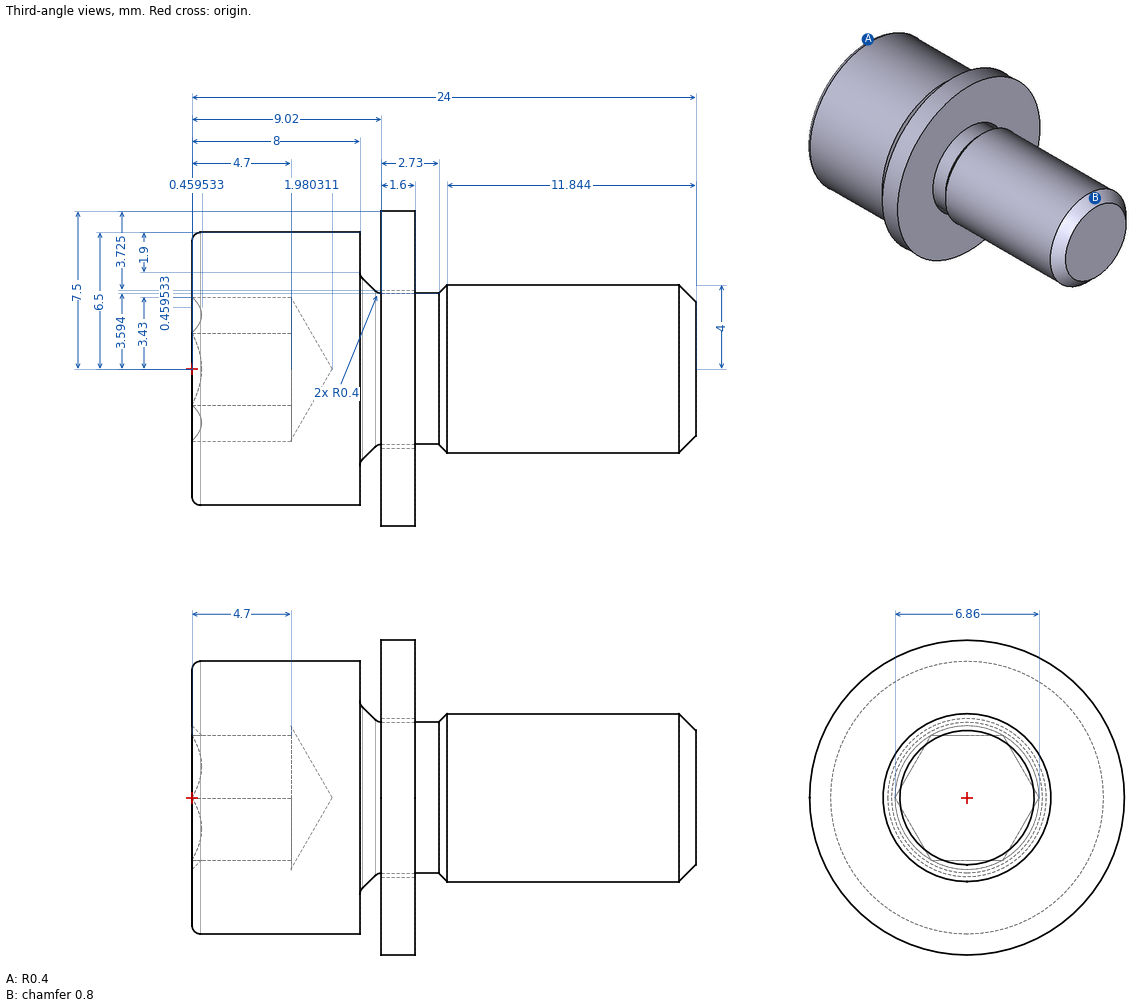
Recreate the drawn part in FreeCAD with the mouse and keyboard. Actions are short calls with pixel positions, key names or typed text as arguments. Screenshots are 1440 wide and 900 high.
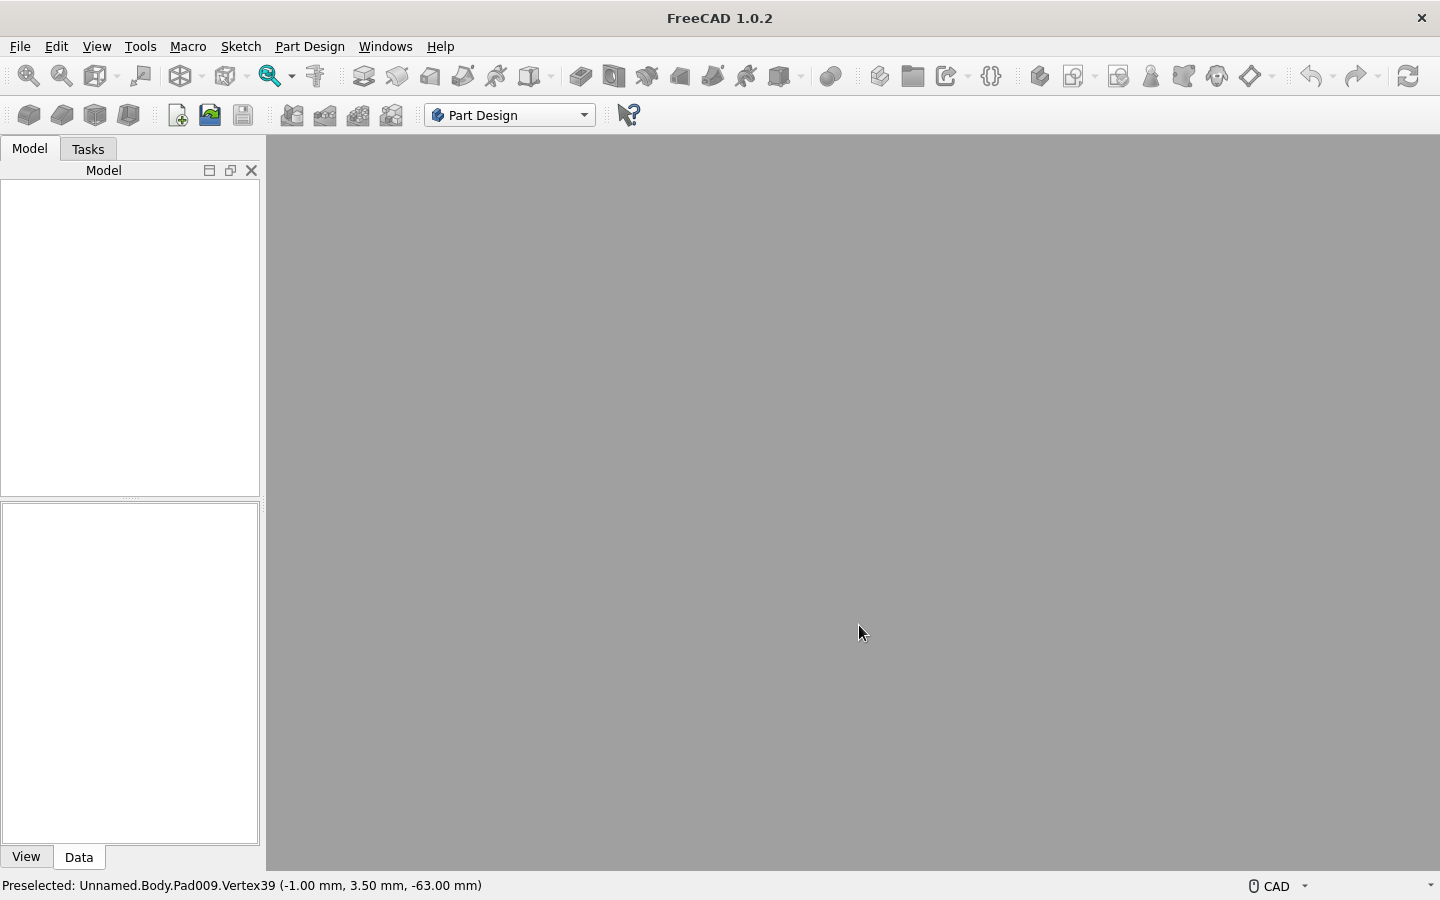
click(177, 116)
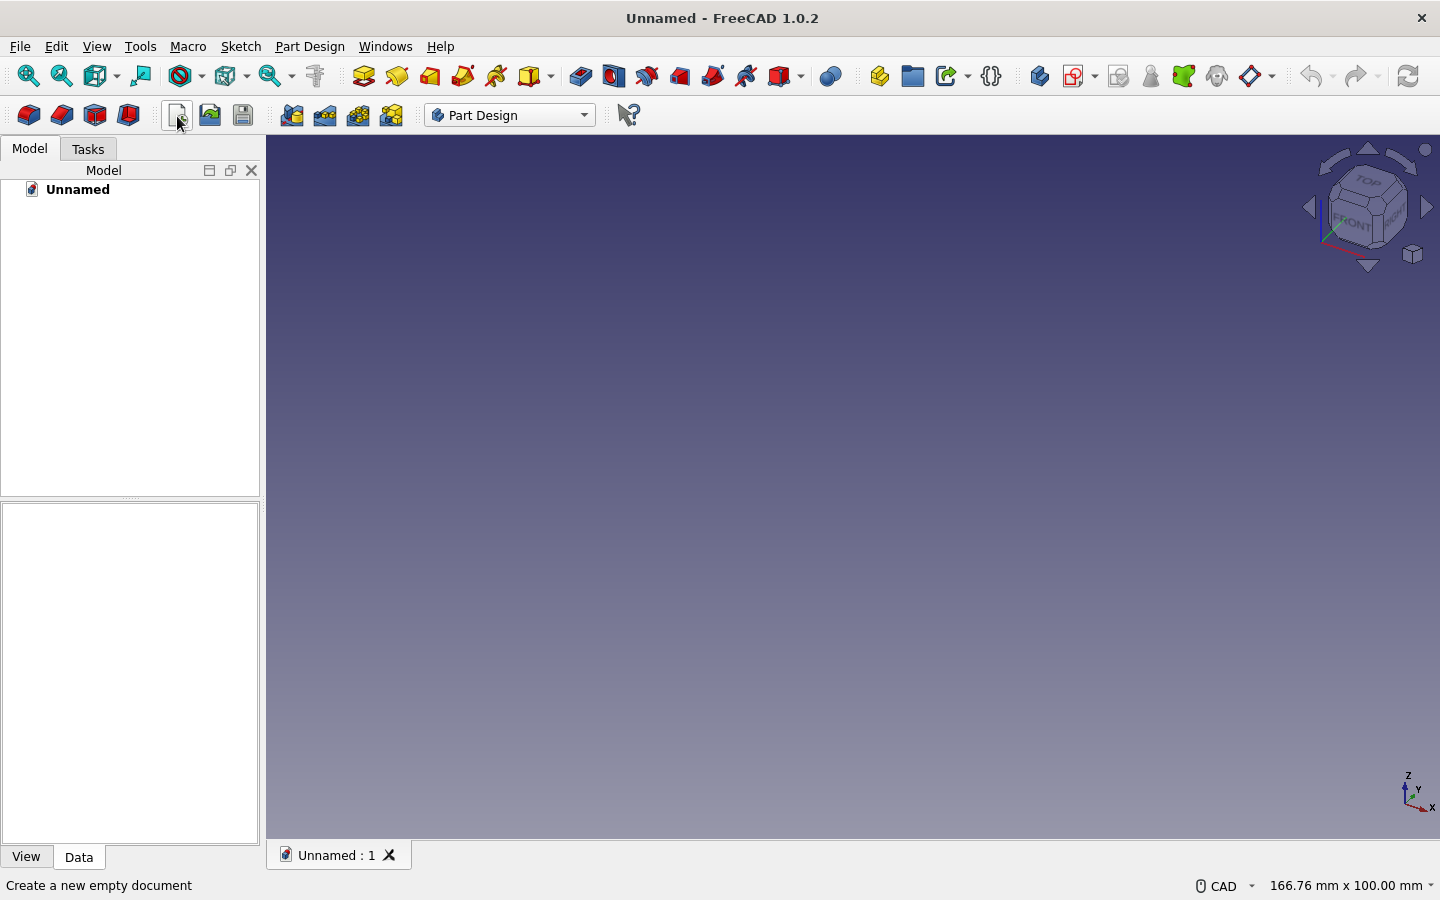
click(1072, 76)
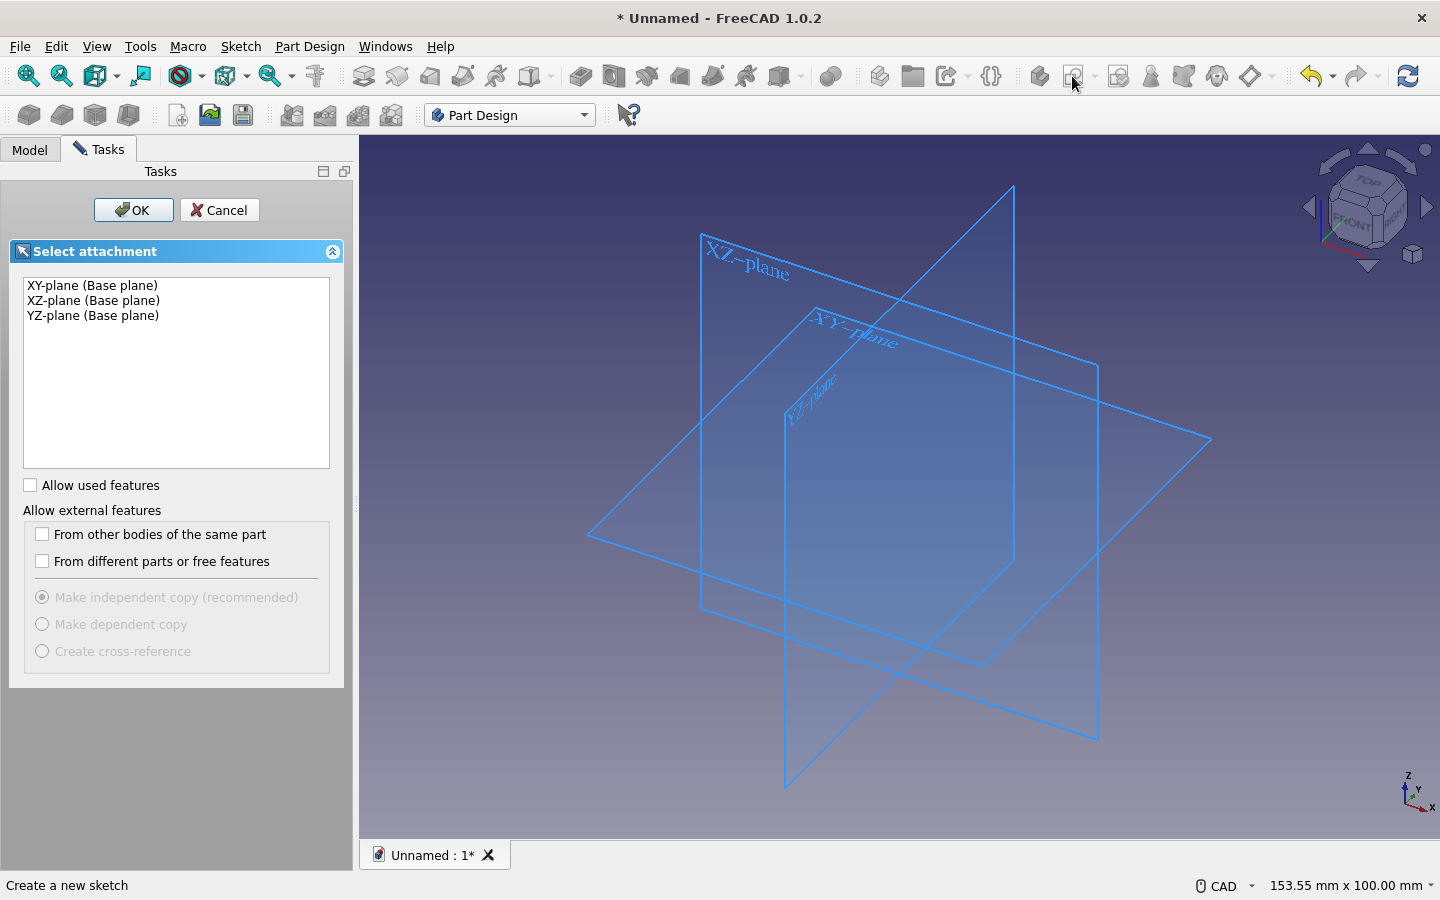
click(84, 286)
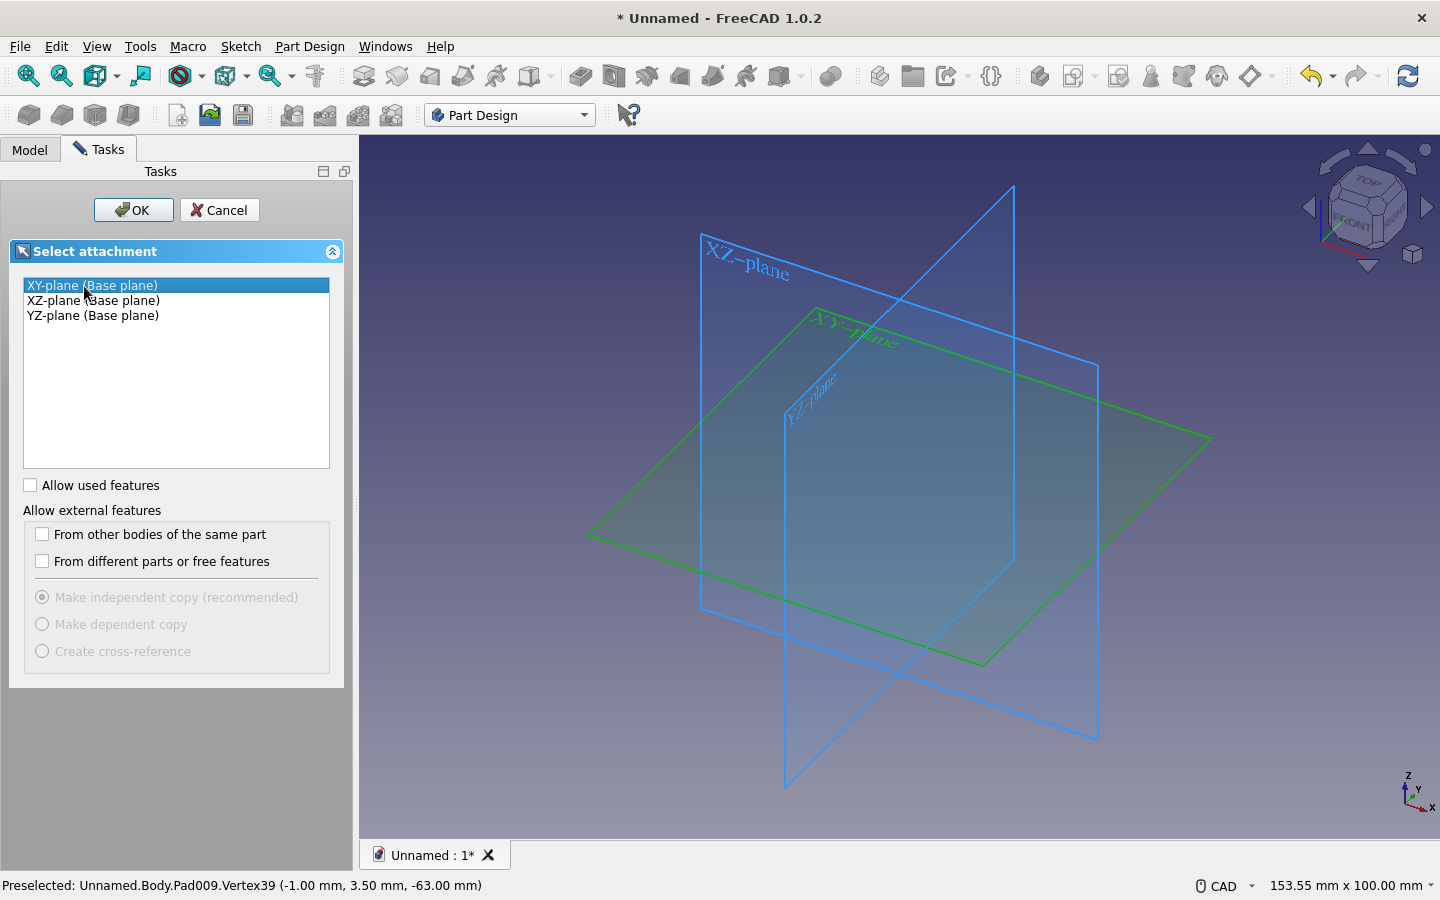
click(134, 210)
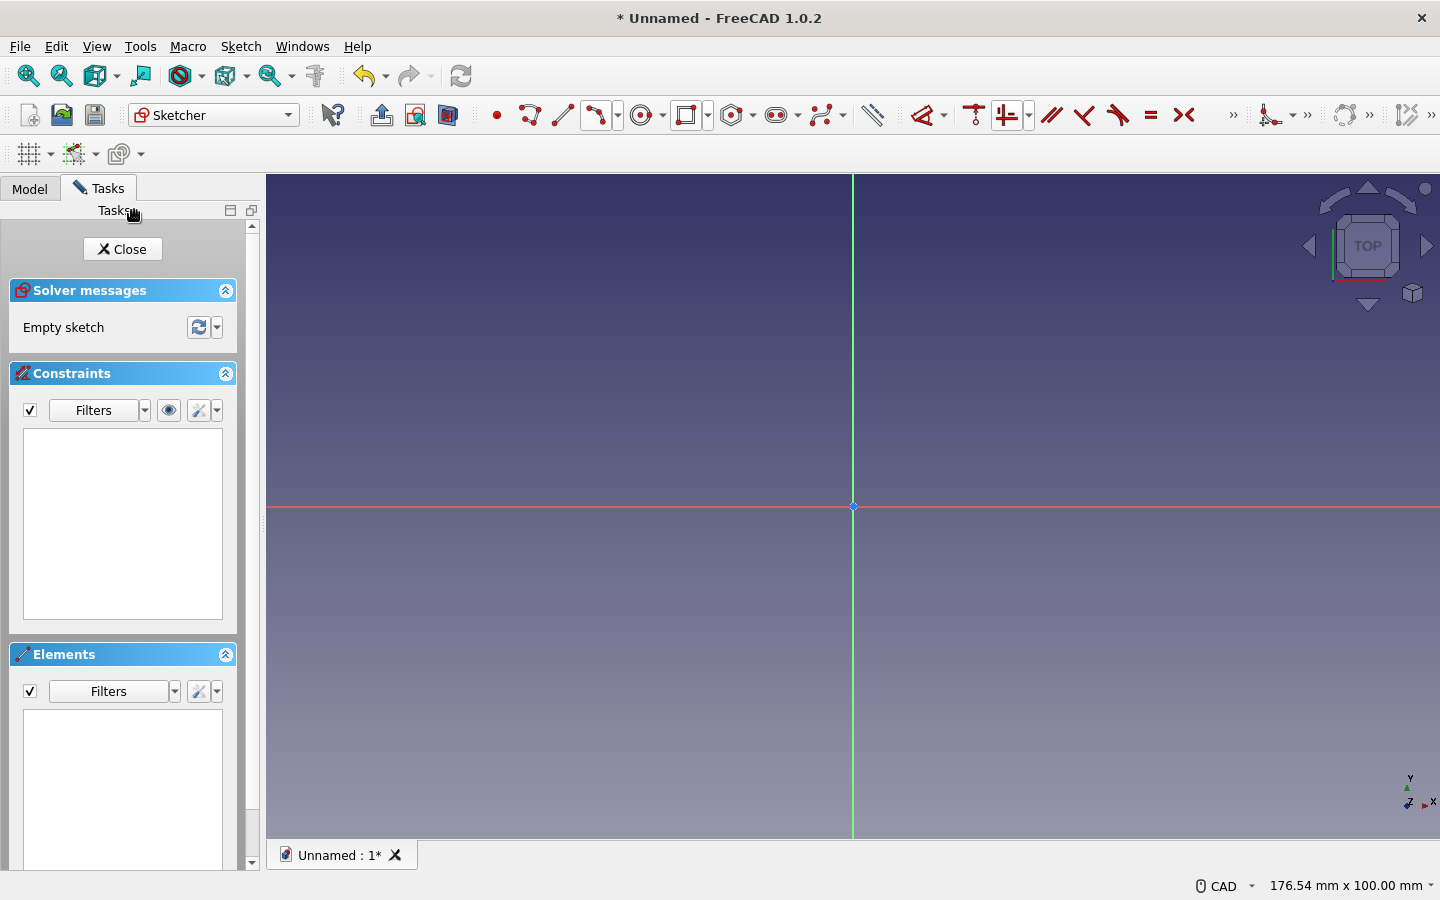
scroll(981, 478, up, 7)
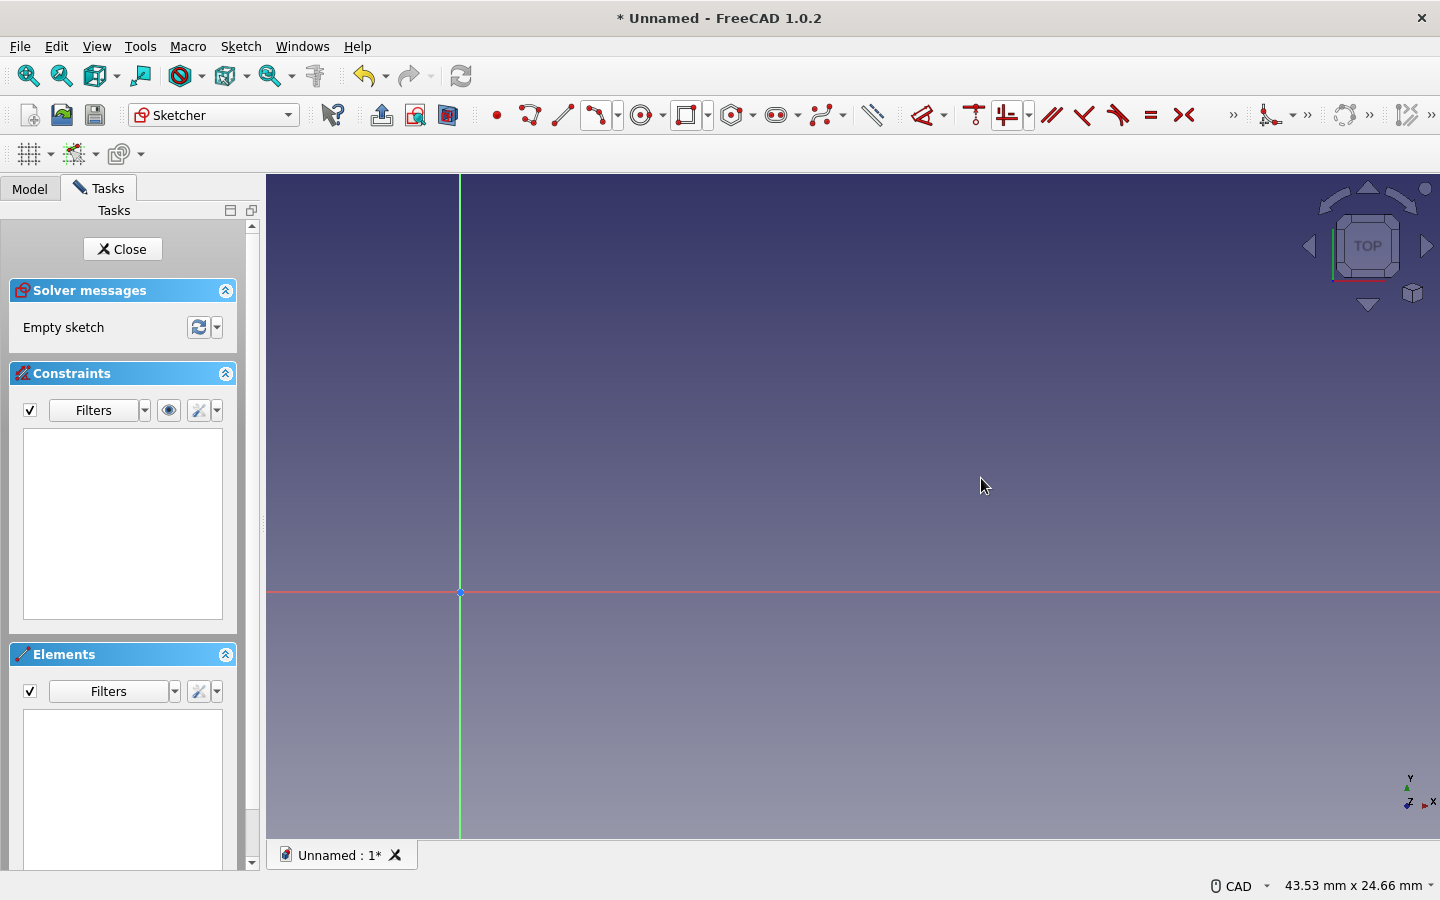
click(563, 116)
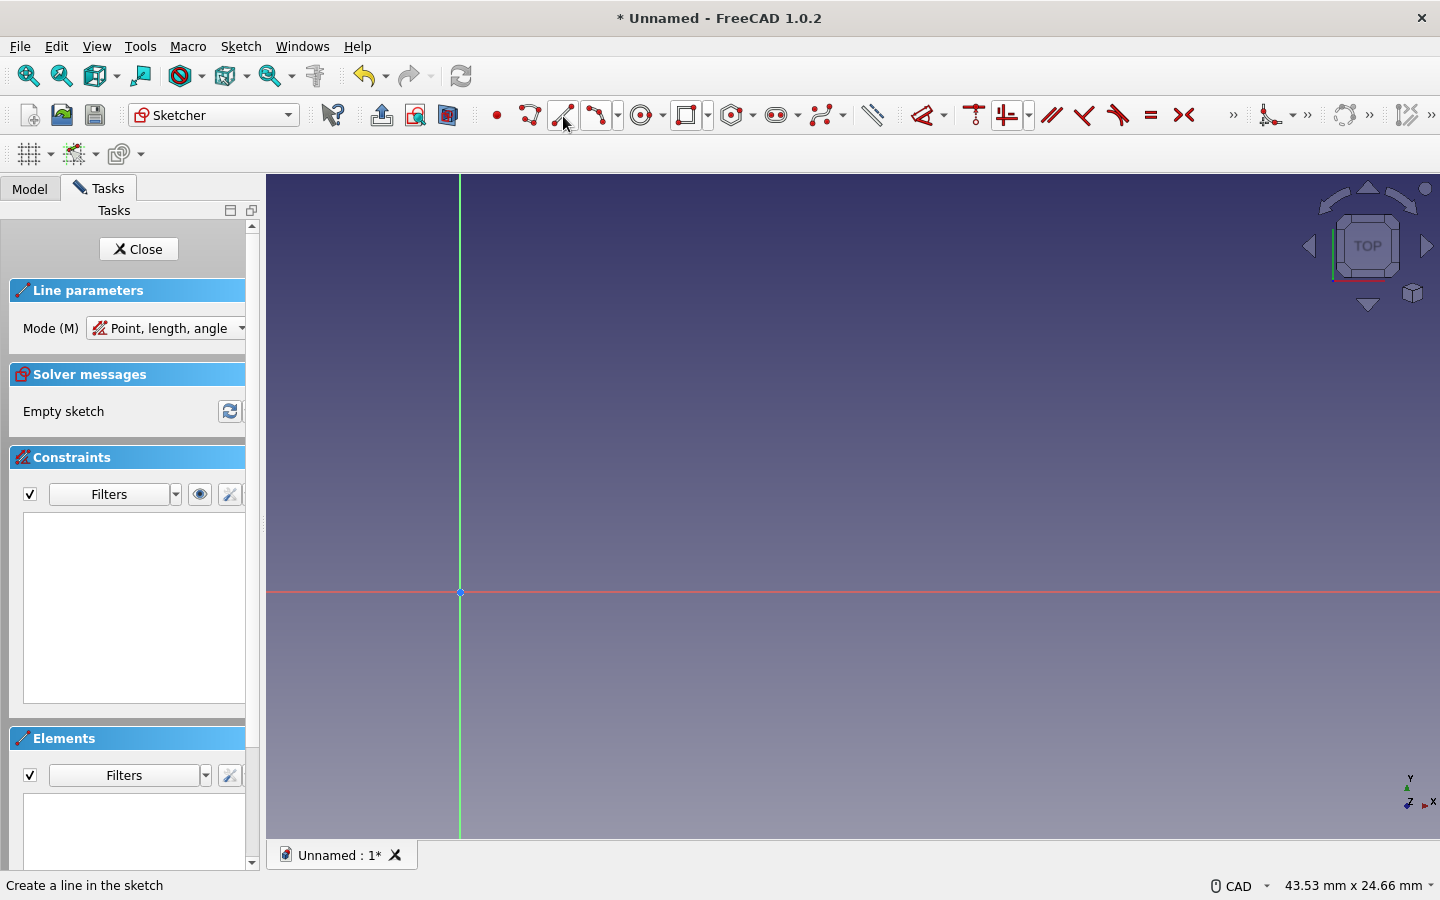
click(696, 492)
click(679, 476)